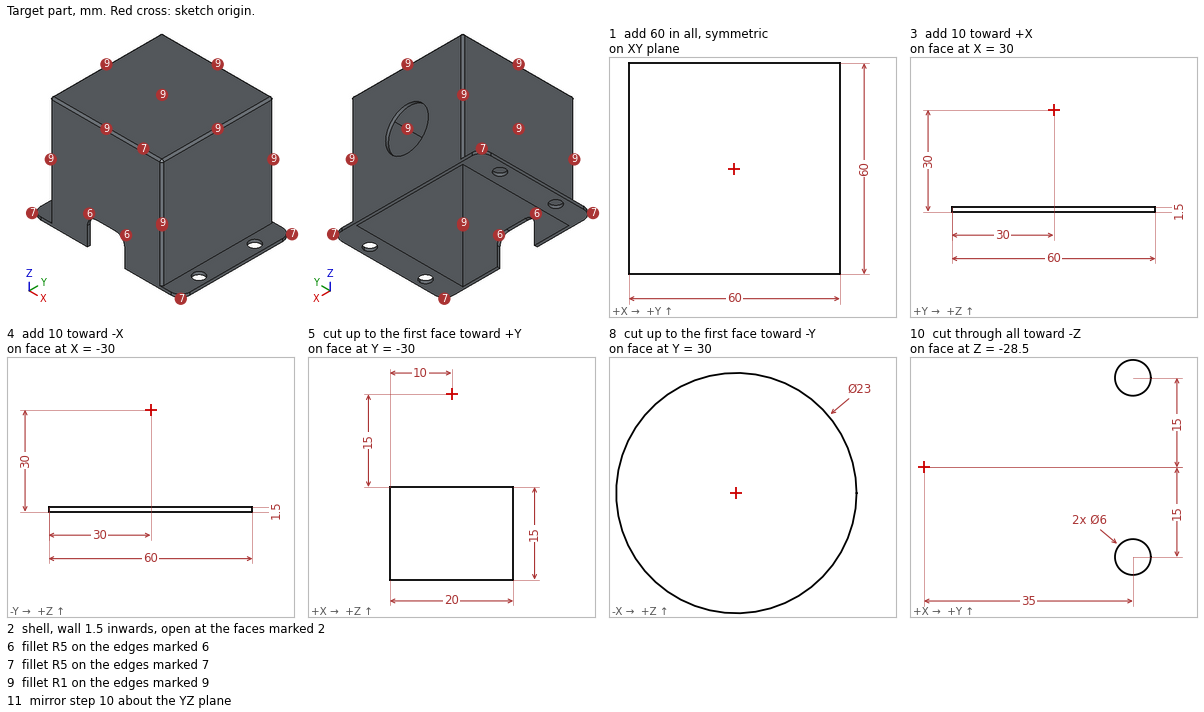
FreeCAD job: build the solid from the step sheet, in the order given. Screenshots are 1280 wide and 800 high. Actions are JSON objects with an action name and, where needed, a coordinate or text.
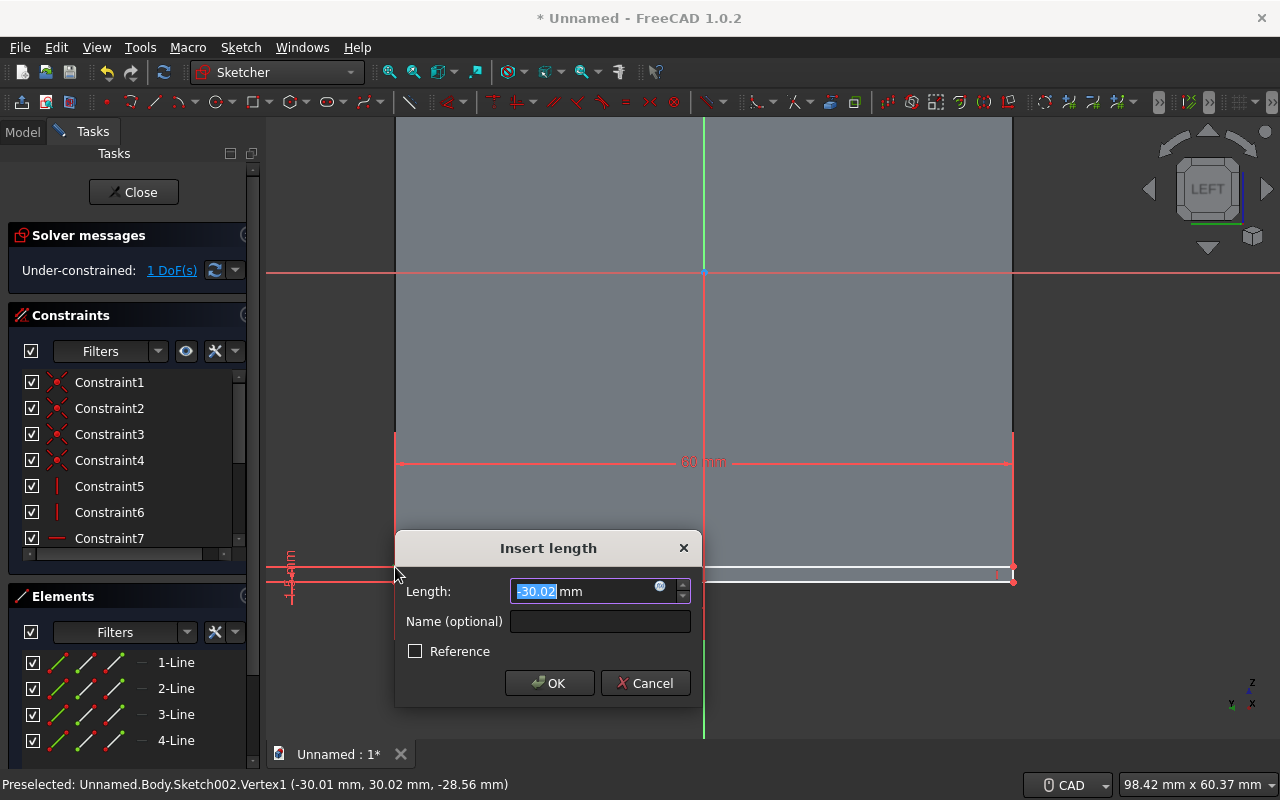
{"action": "type", "text": "-30"}
{"action": "key", "text": "Return"}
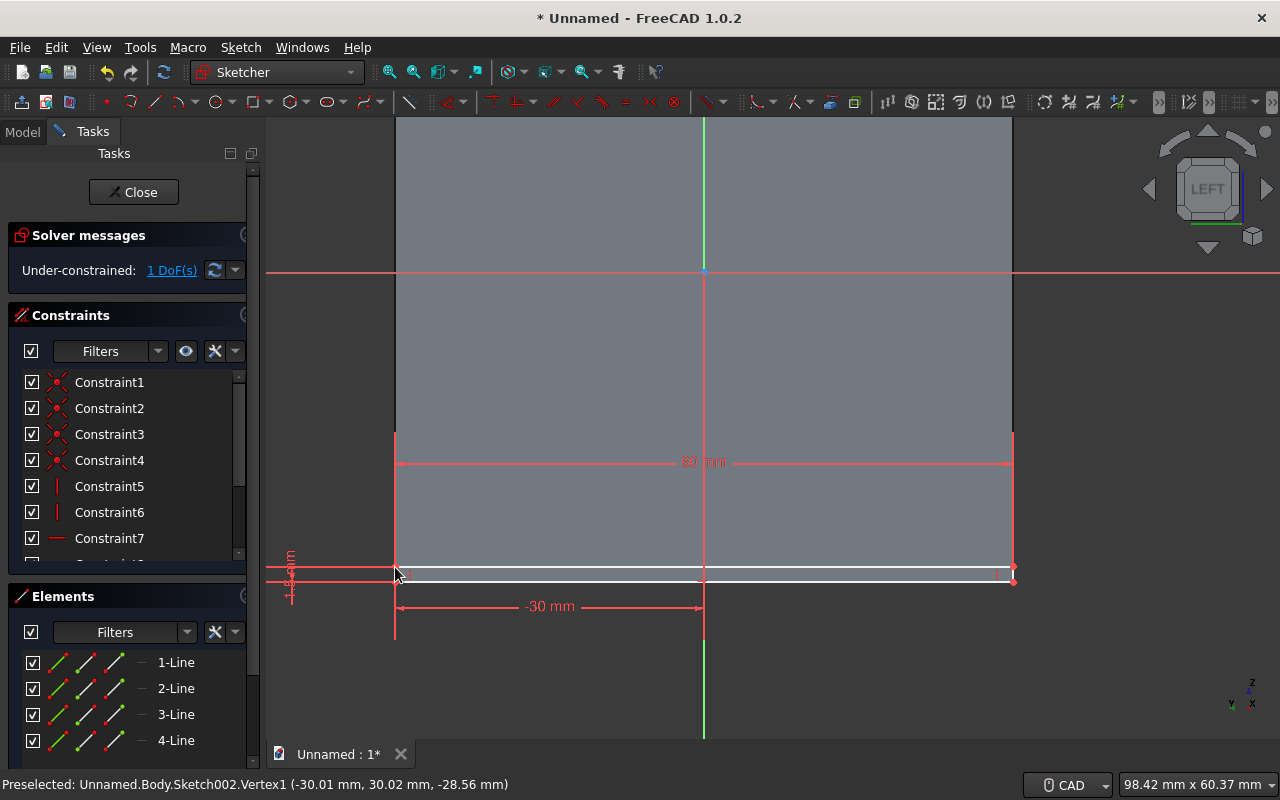
{"action": "left_click", "coordinate": [395, 582]}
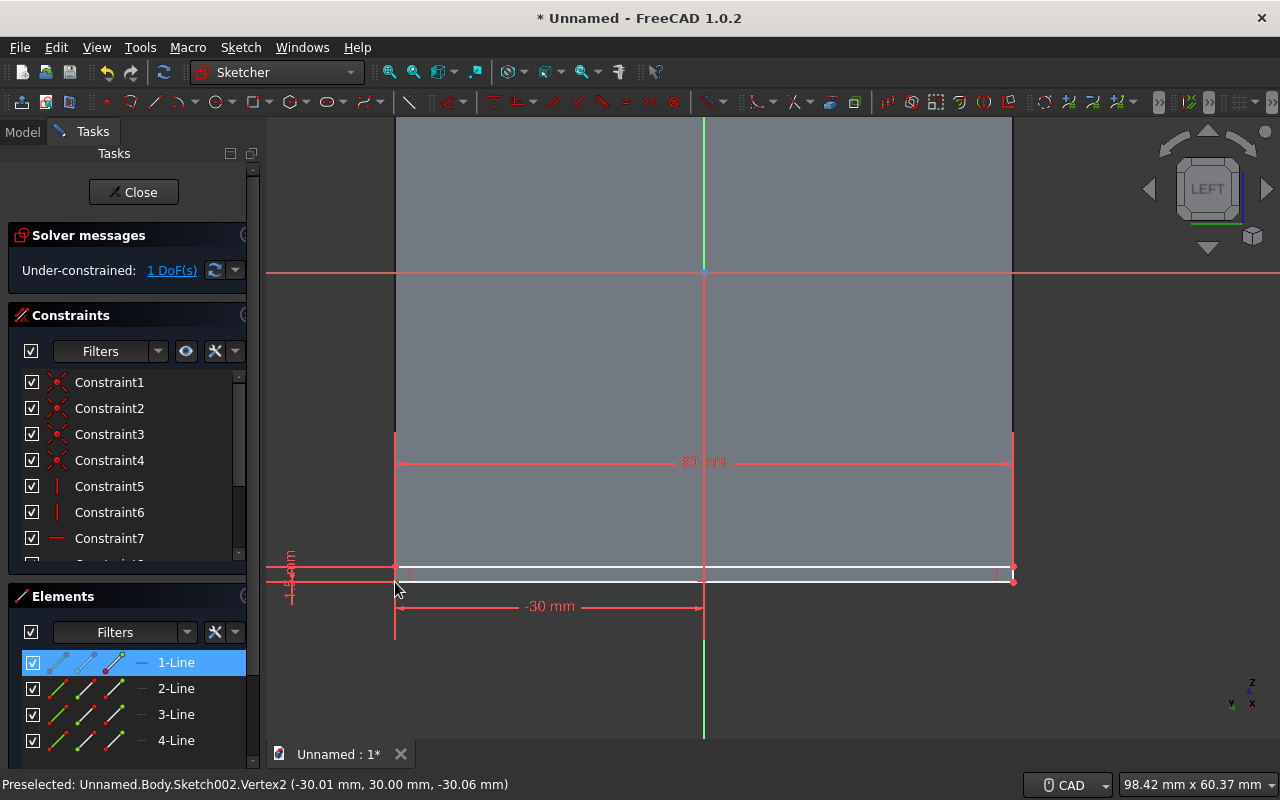
{"action": "key", "text": "i"}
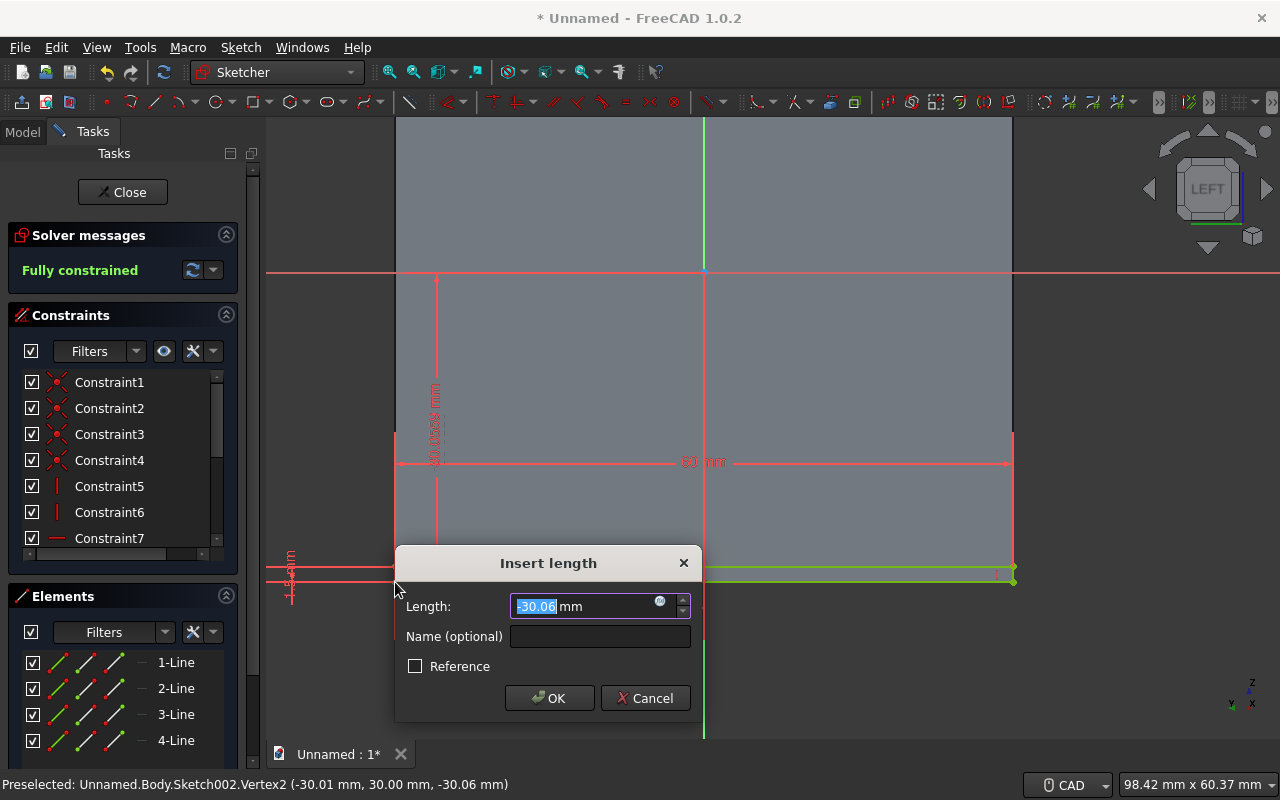
{"action": "type", "text": "-30"}
{"action": "key", "text": "Return"}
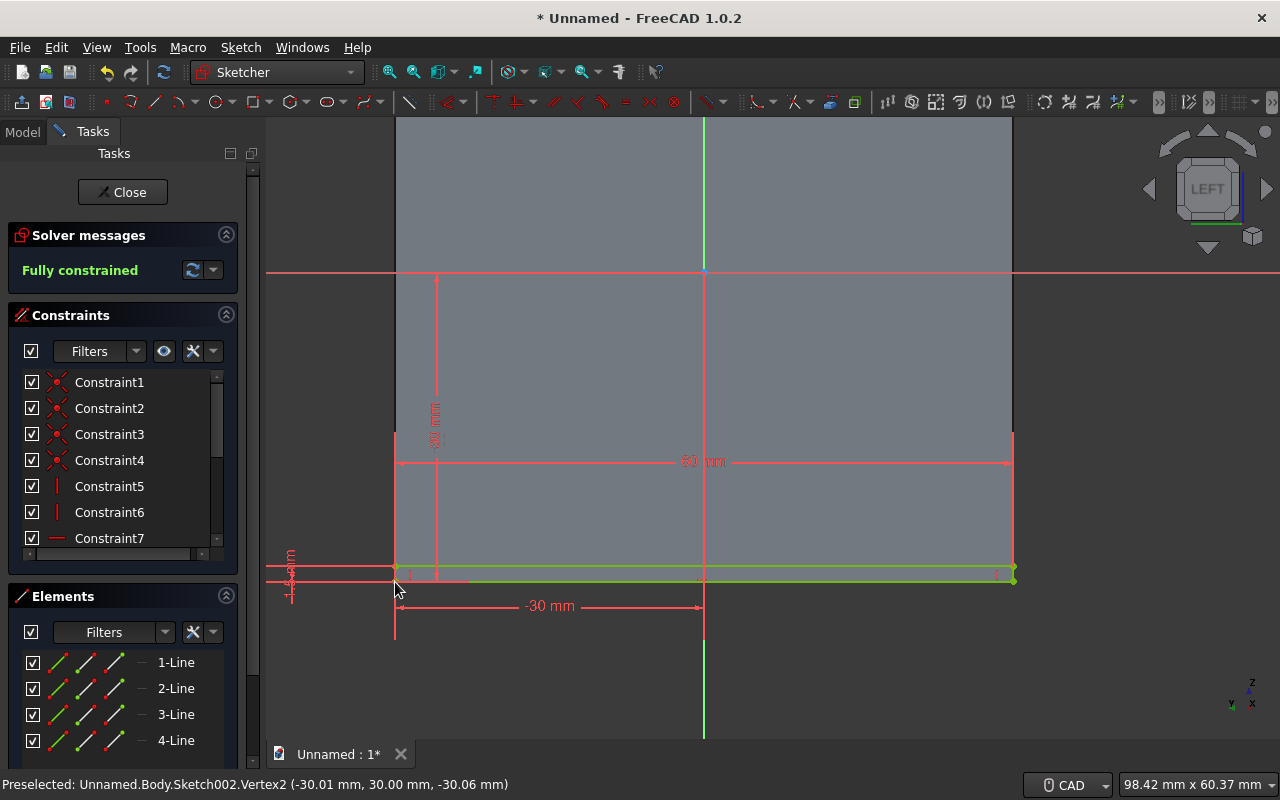
{"action": "left_click", "coordinate": [123, 192]}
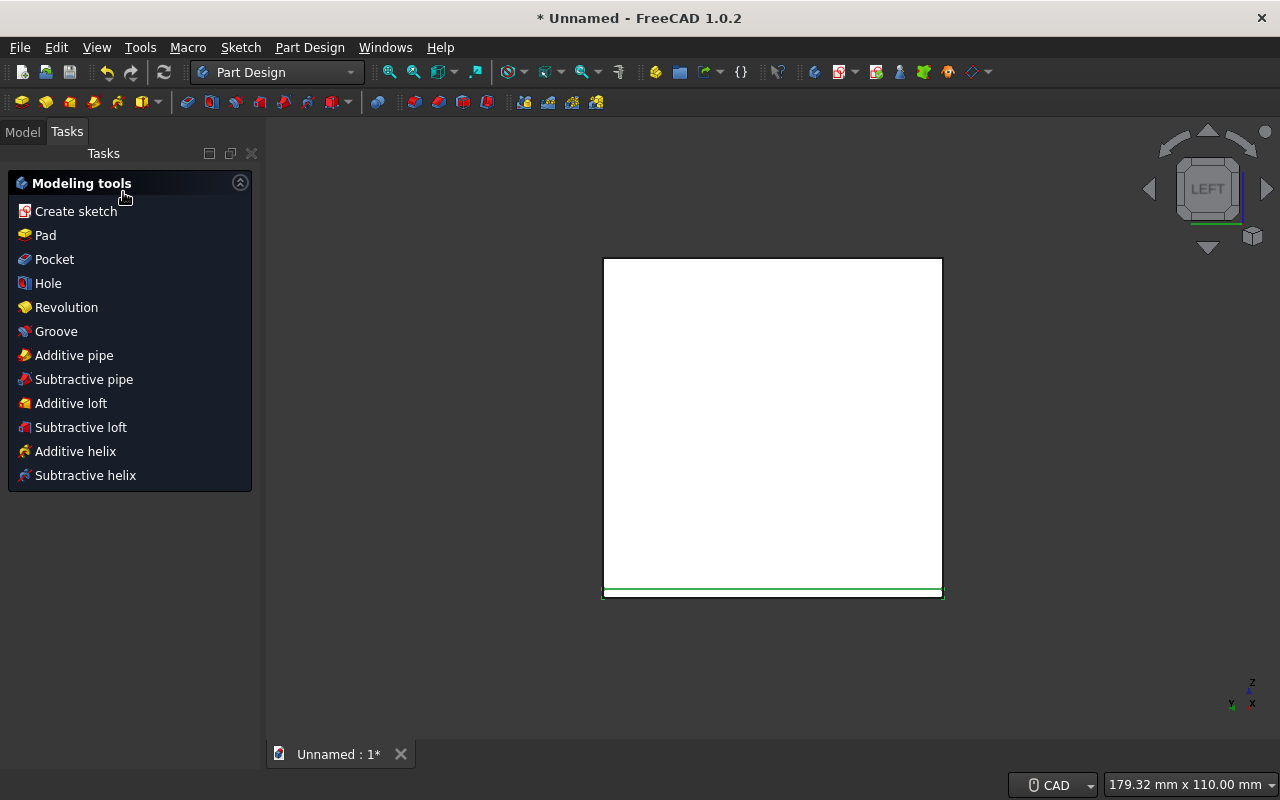
{"action": "left_click", "coordinate": [22, 102]}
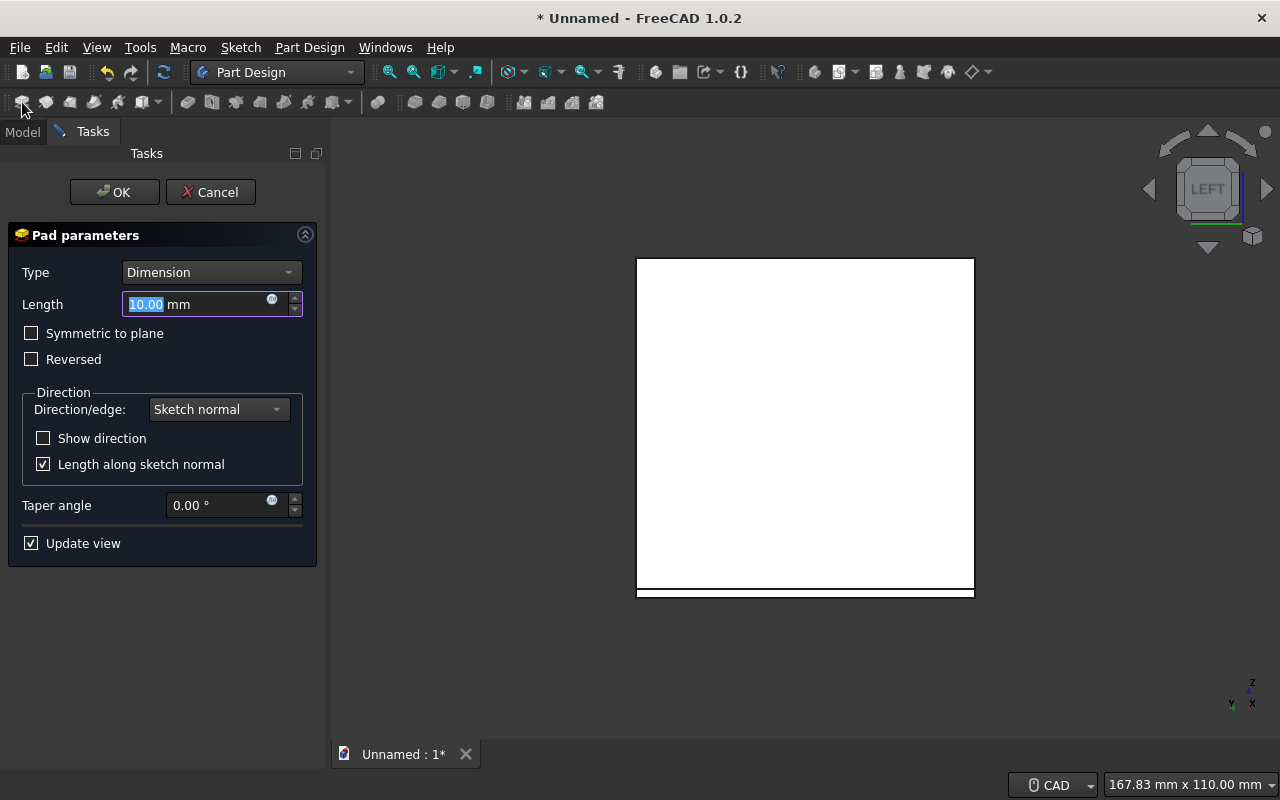
{"action": "type", "text": "10"}
{"action": "key", "text": "Tab"}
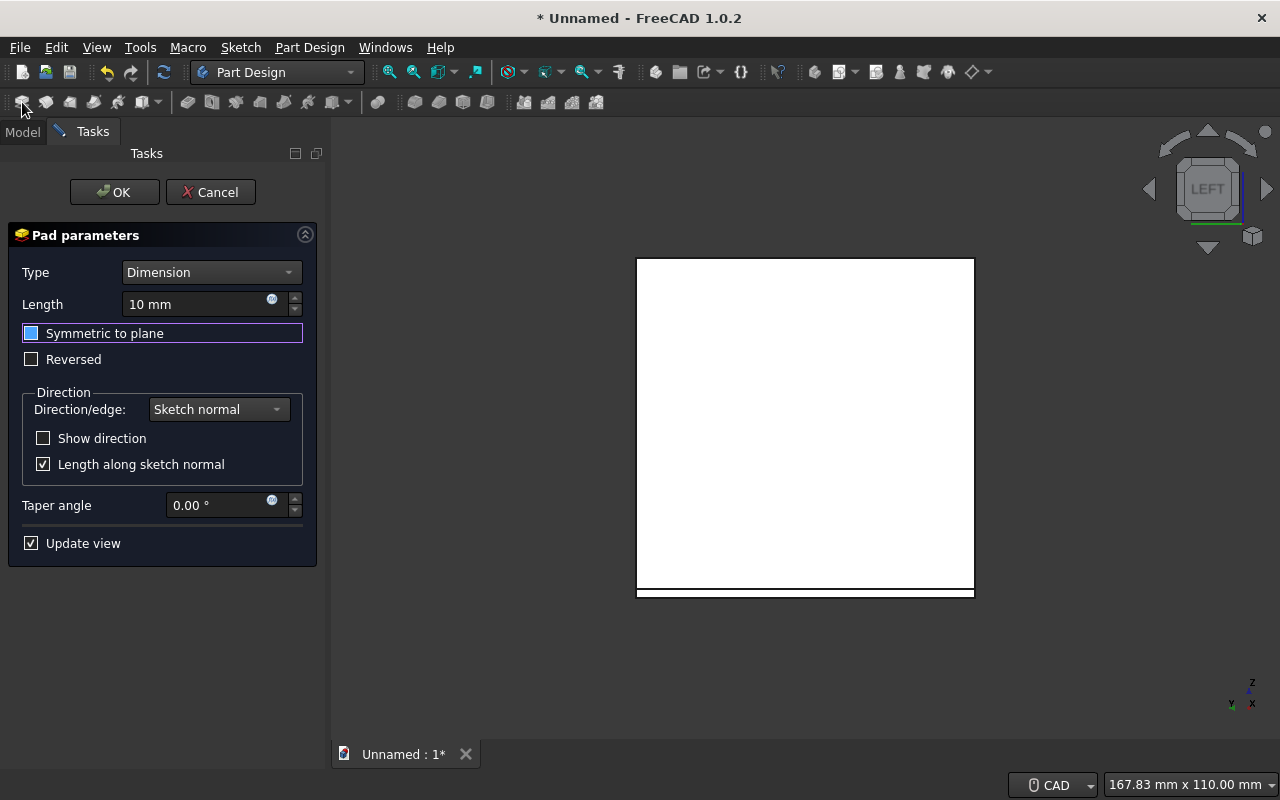
{"action": "left_click", "coordinate": [115, 192]}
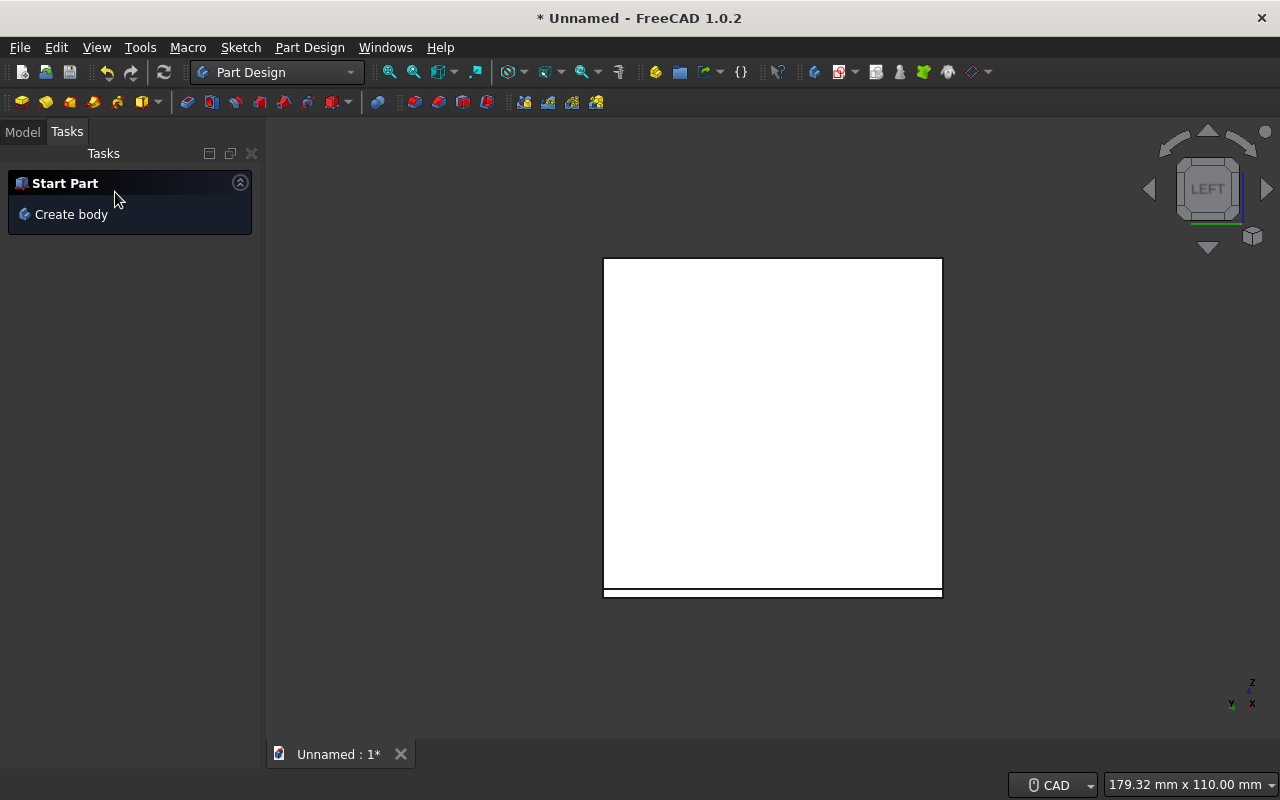
{"action": "key", "text": "0"}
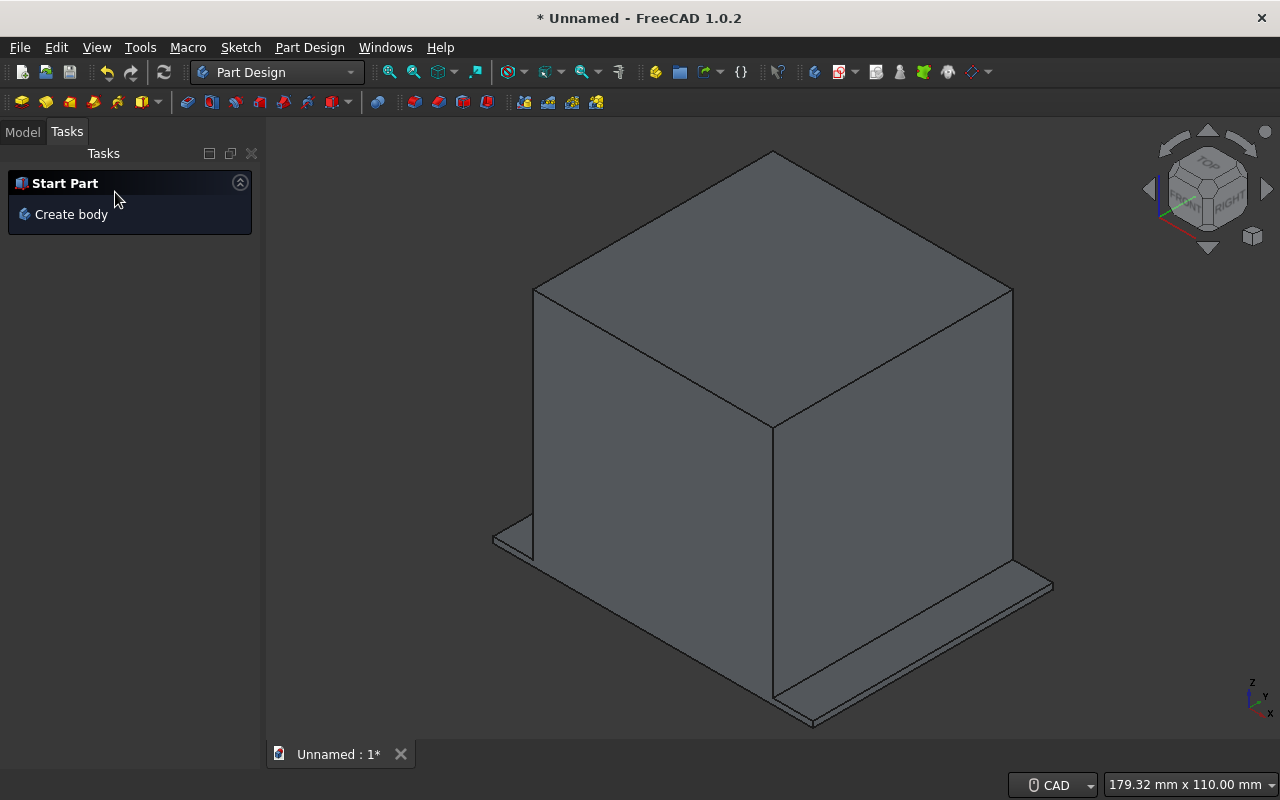
{"action": "left_click", "coordinate": [653, 496]}